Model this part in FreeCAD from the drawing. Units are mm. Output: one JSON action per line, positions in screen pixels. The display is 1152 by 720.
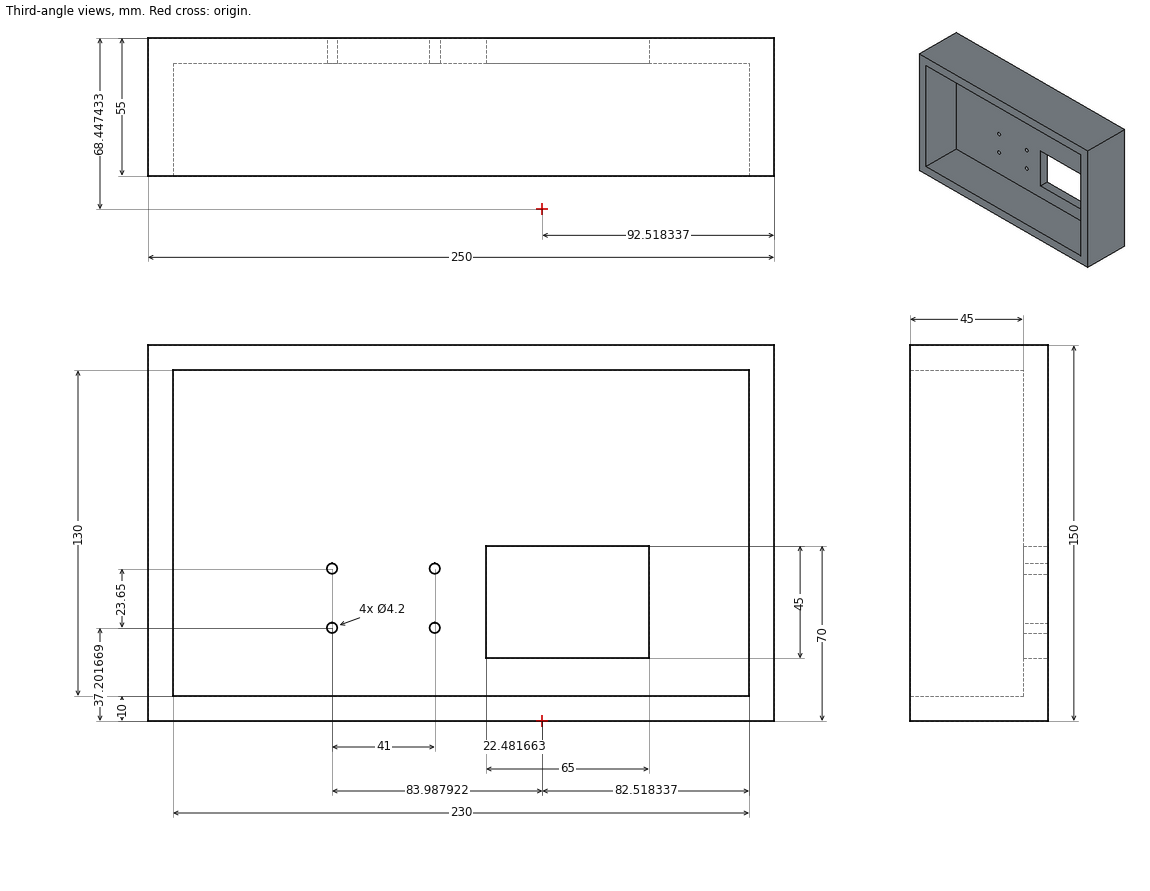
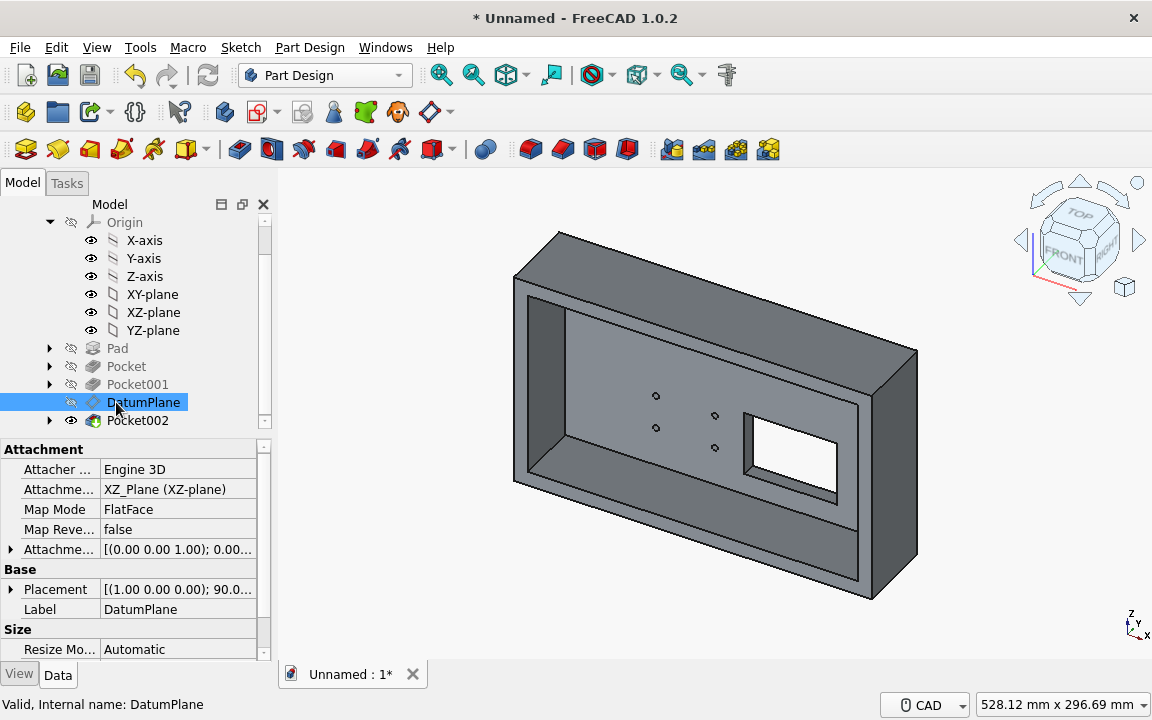
{"action": "key", "text": "0"}